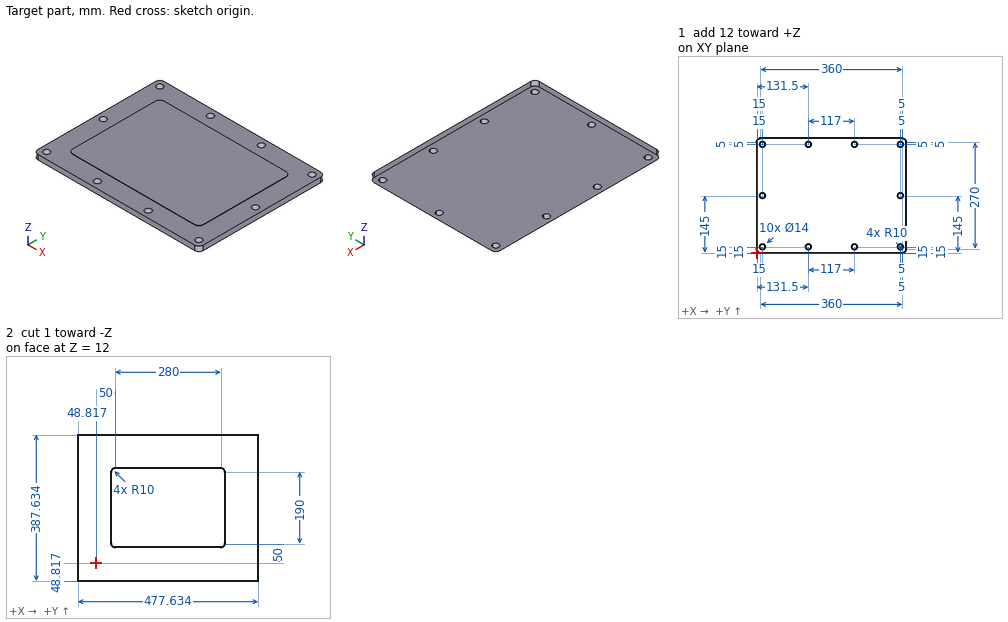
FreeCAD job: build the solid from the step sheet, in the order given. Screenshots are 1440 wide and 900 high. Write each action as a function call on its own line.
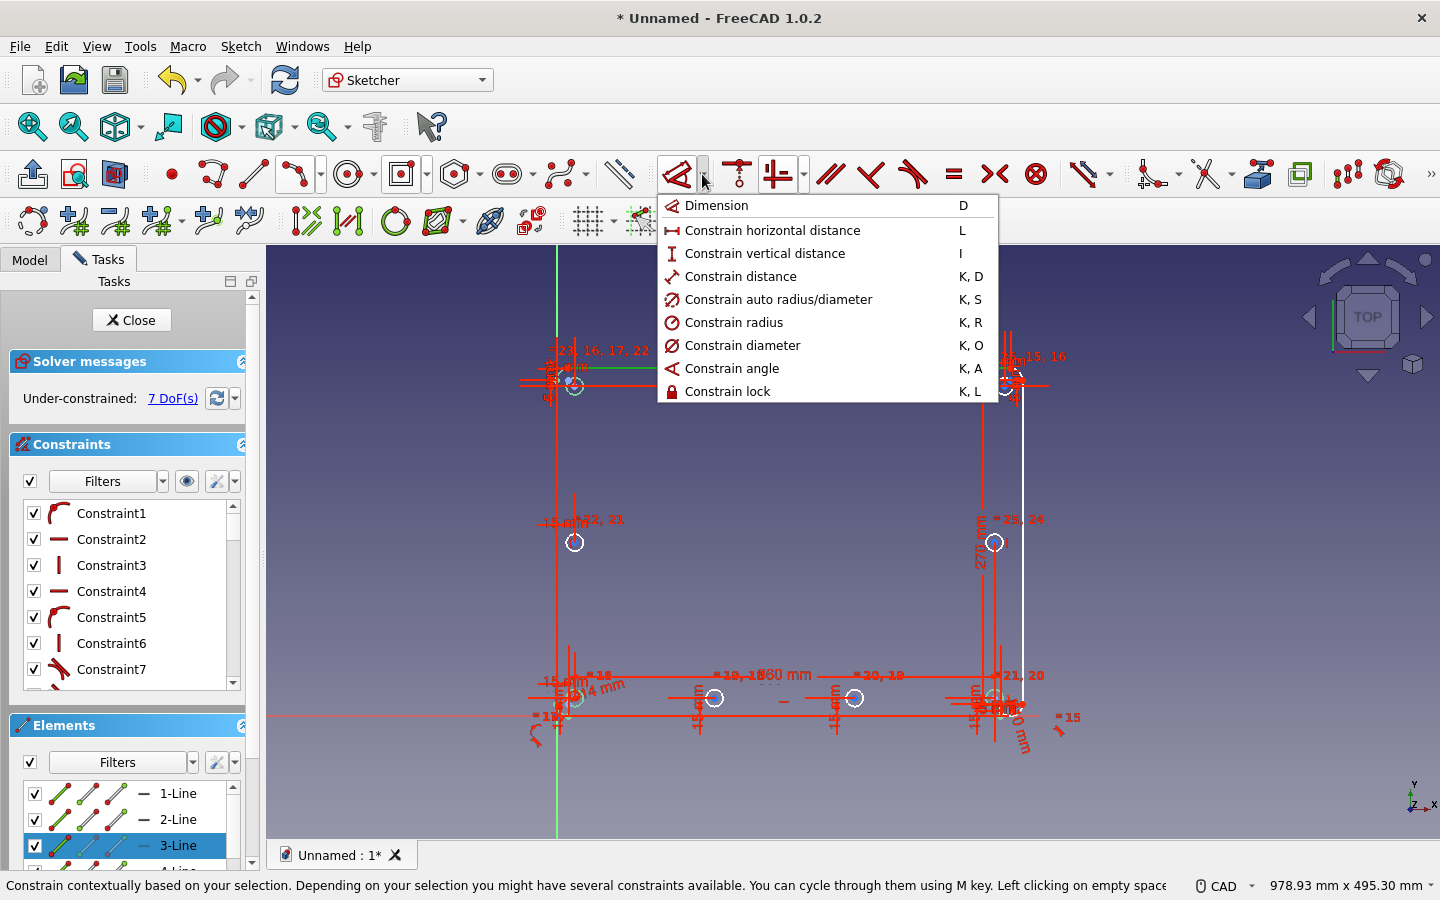
click(828, 230)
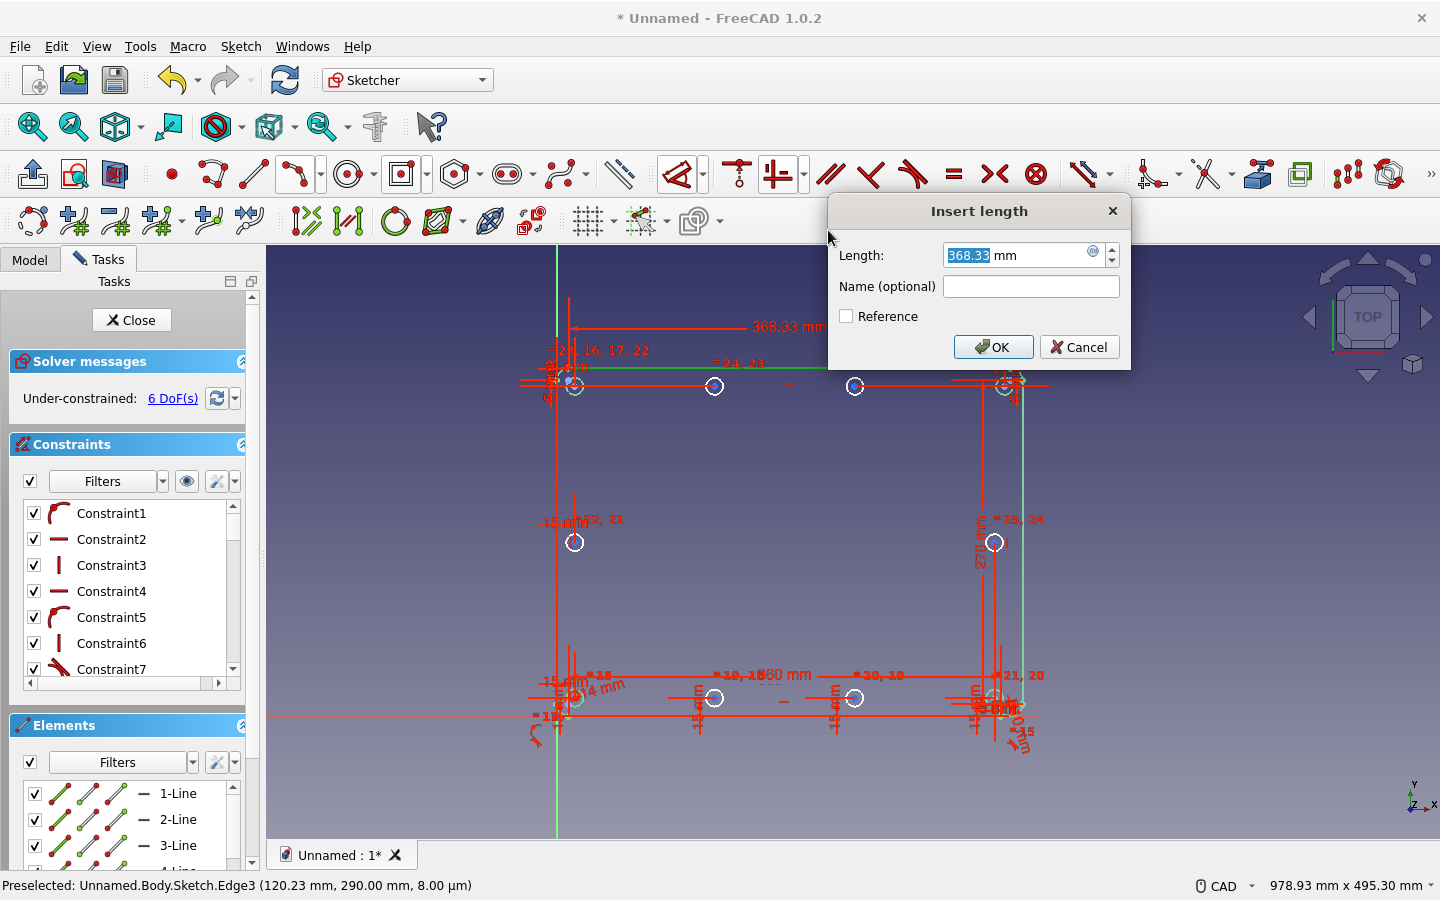
text(360)
key(Return)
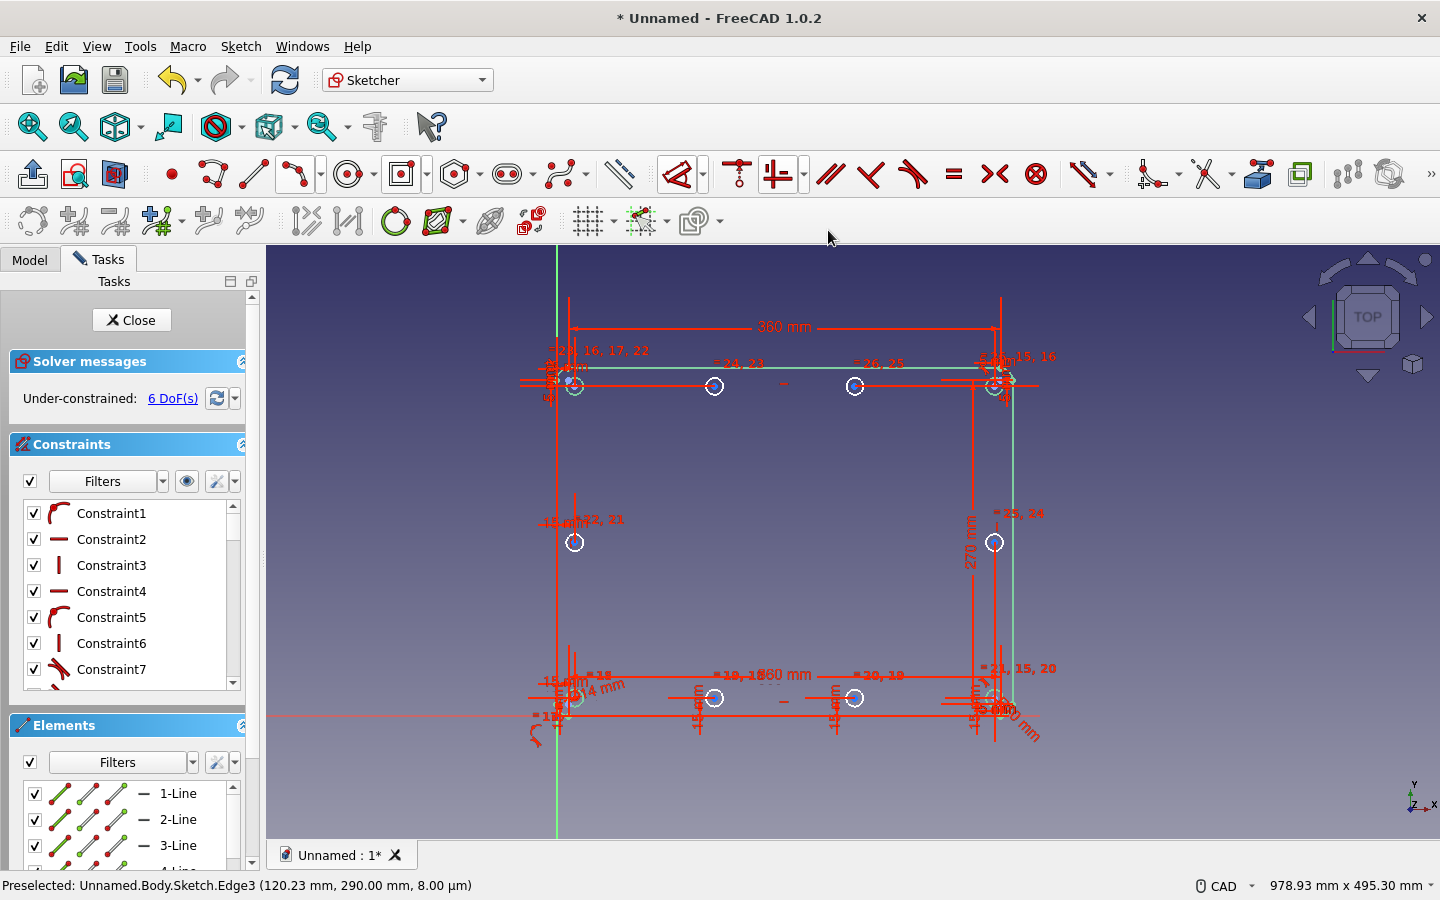
click(575, 543)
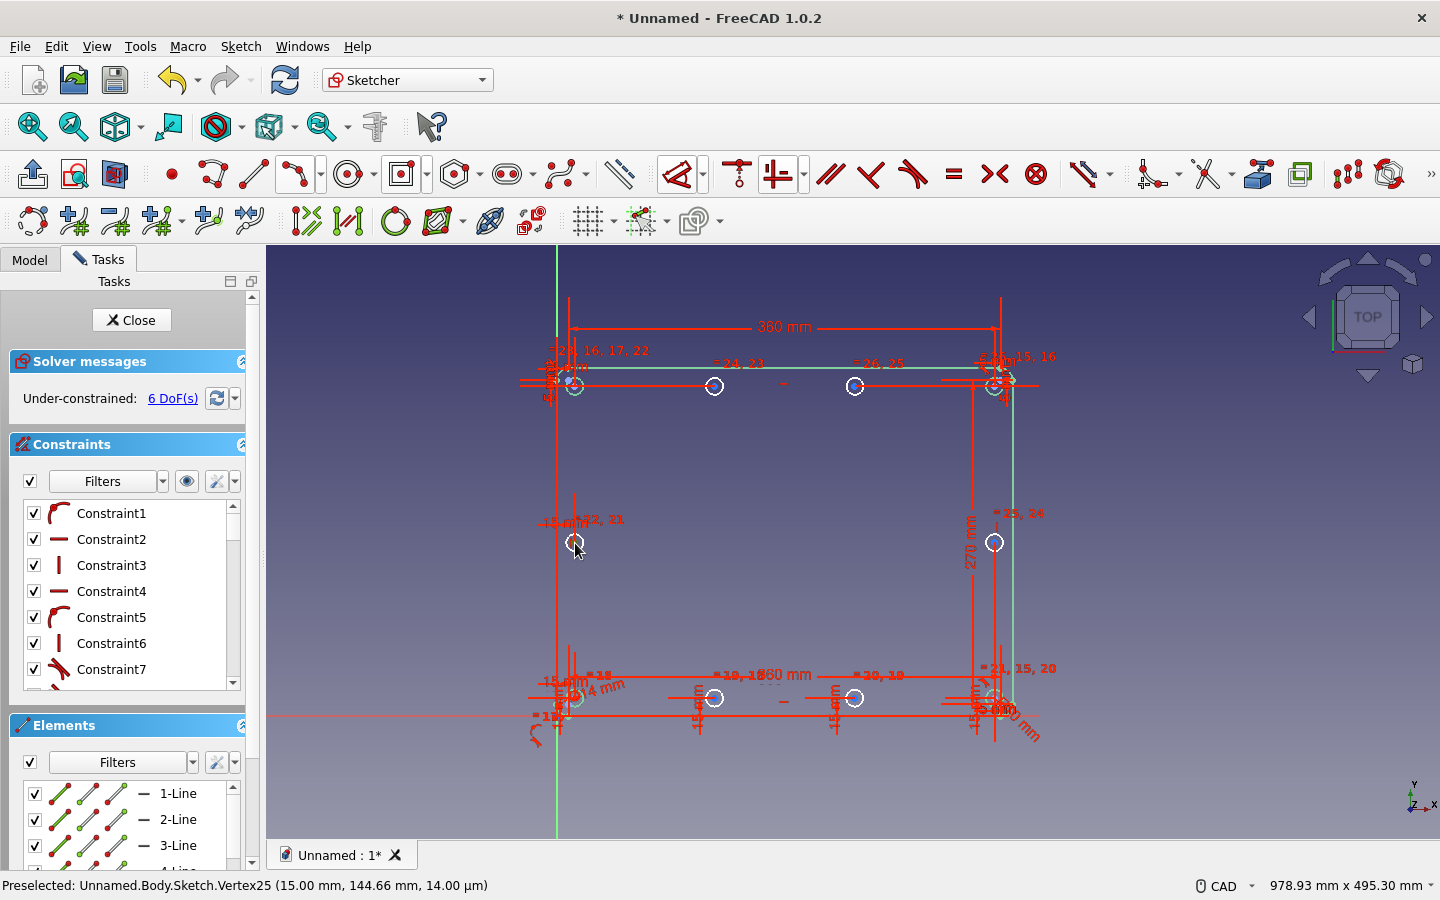
key(i)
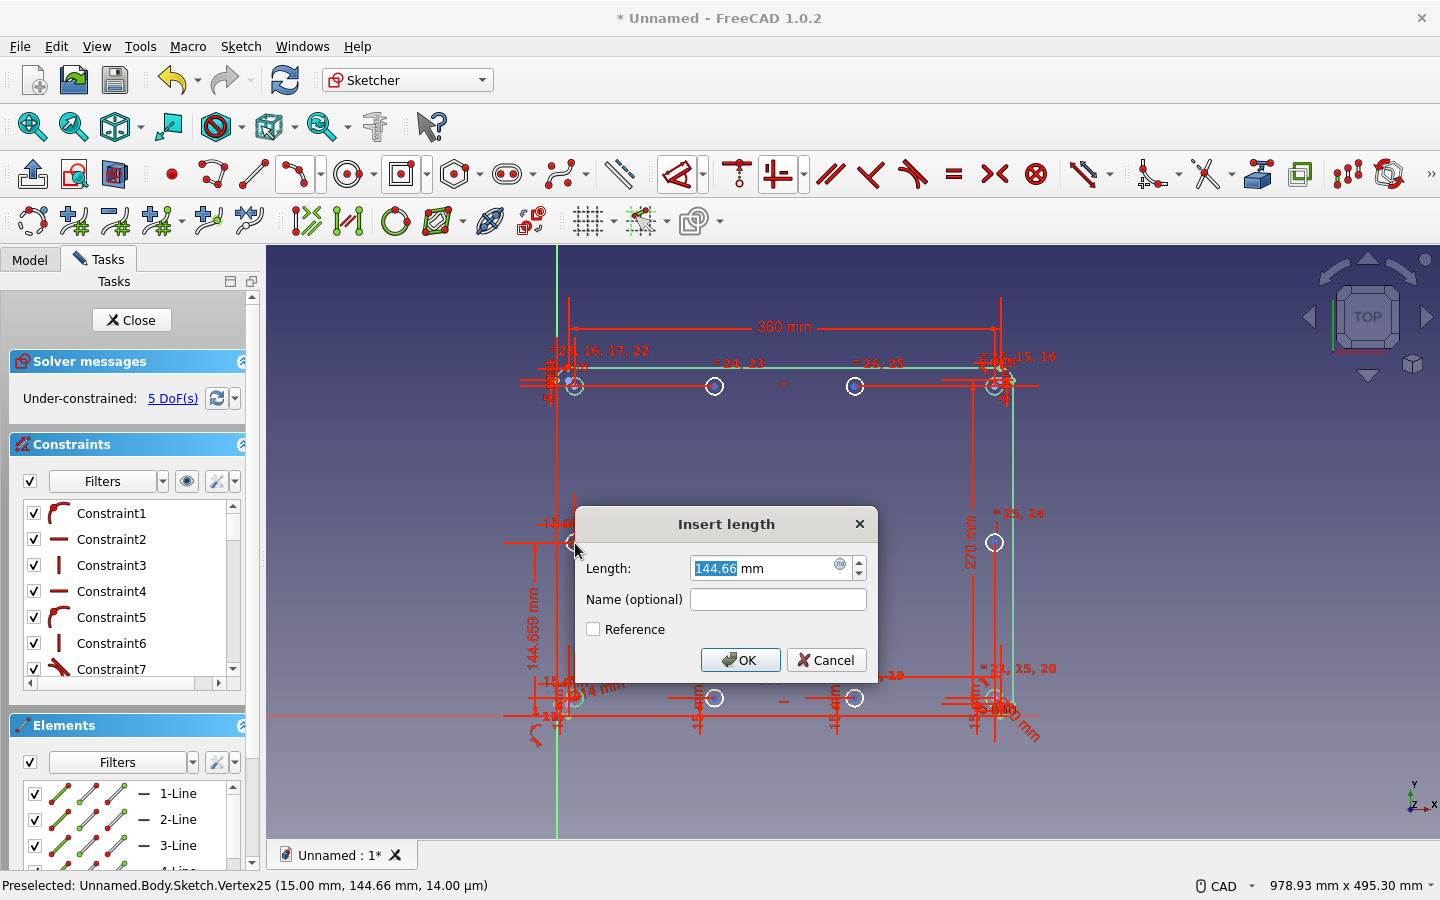
text(145)
key(Return)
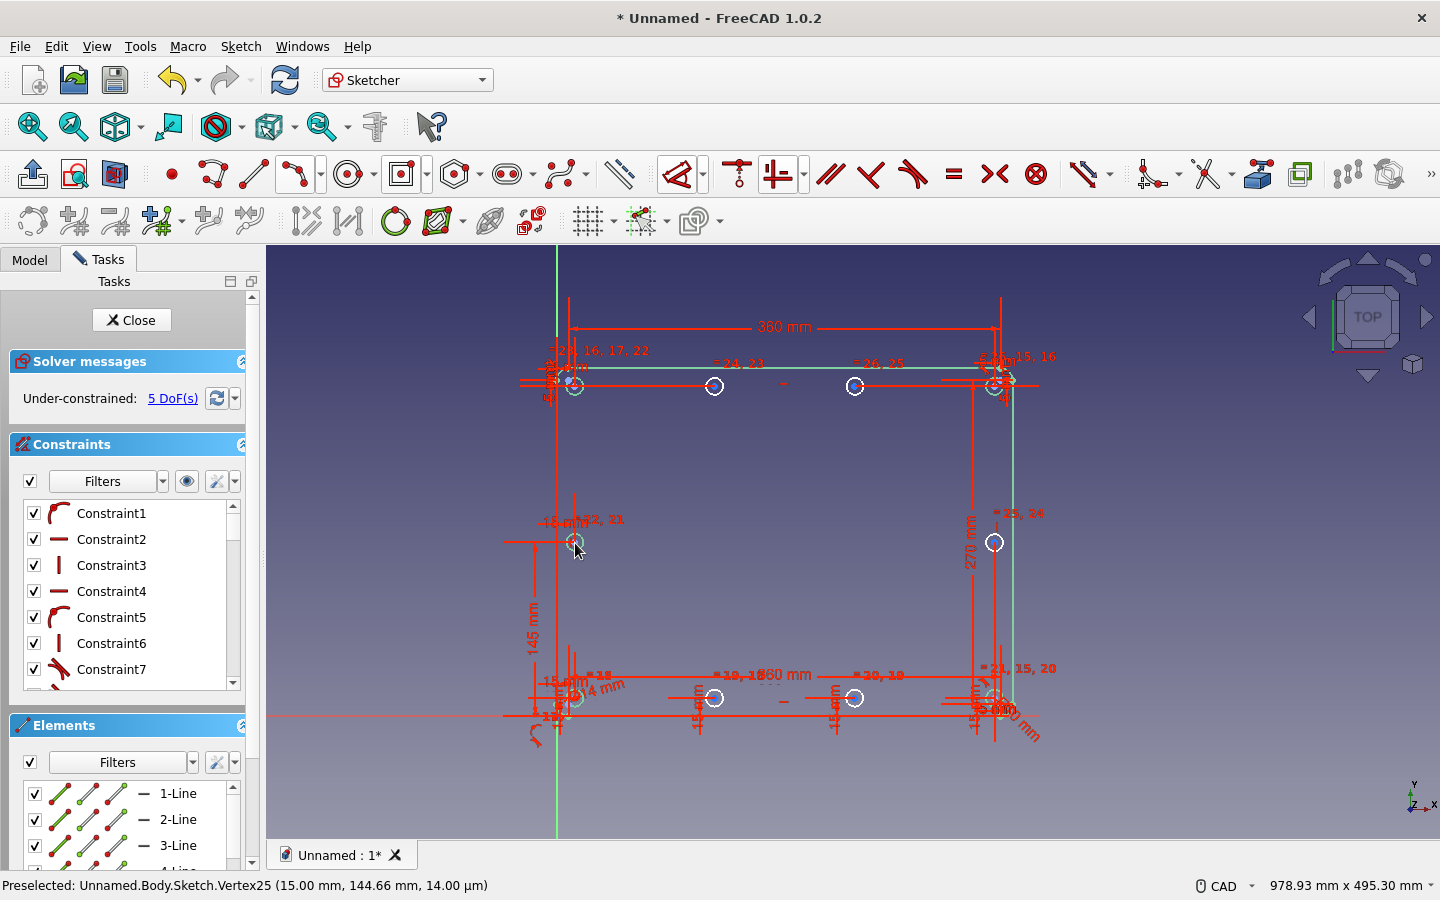
click(995, 543)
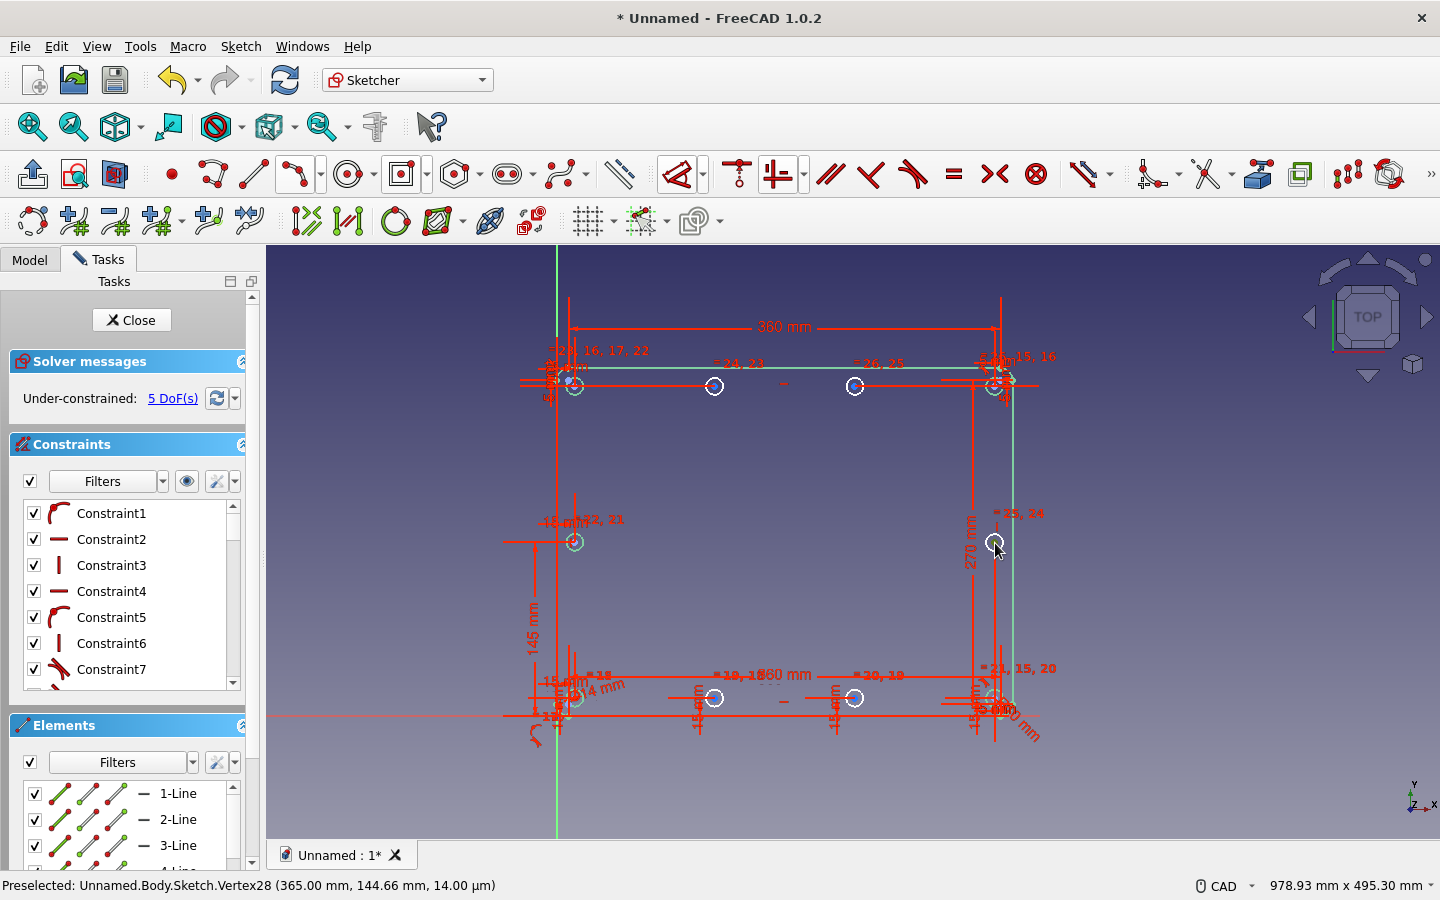
key(i)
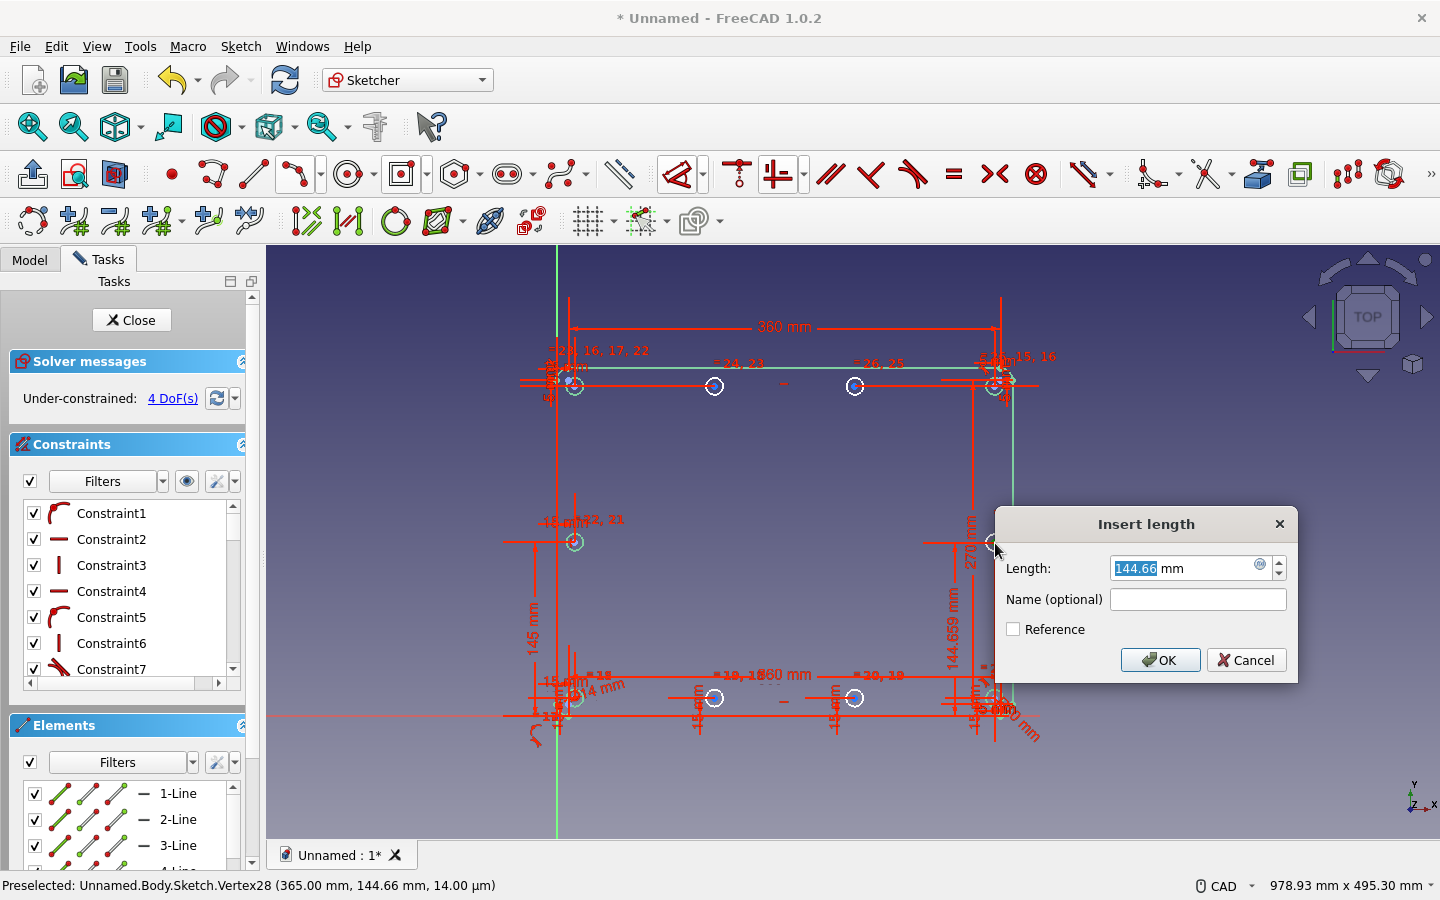
text(145)
key(Return)